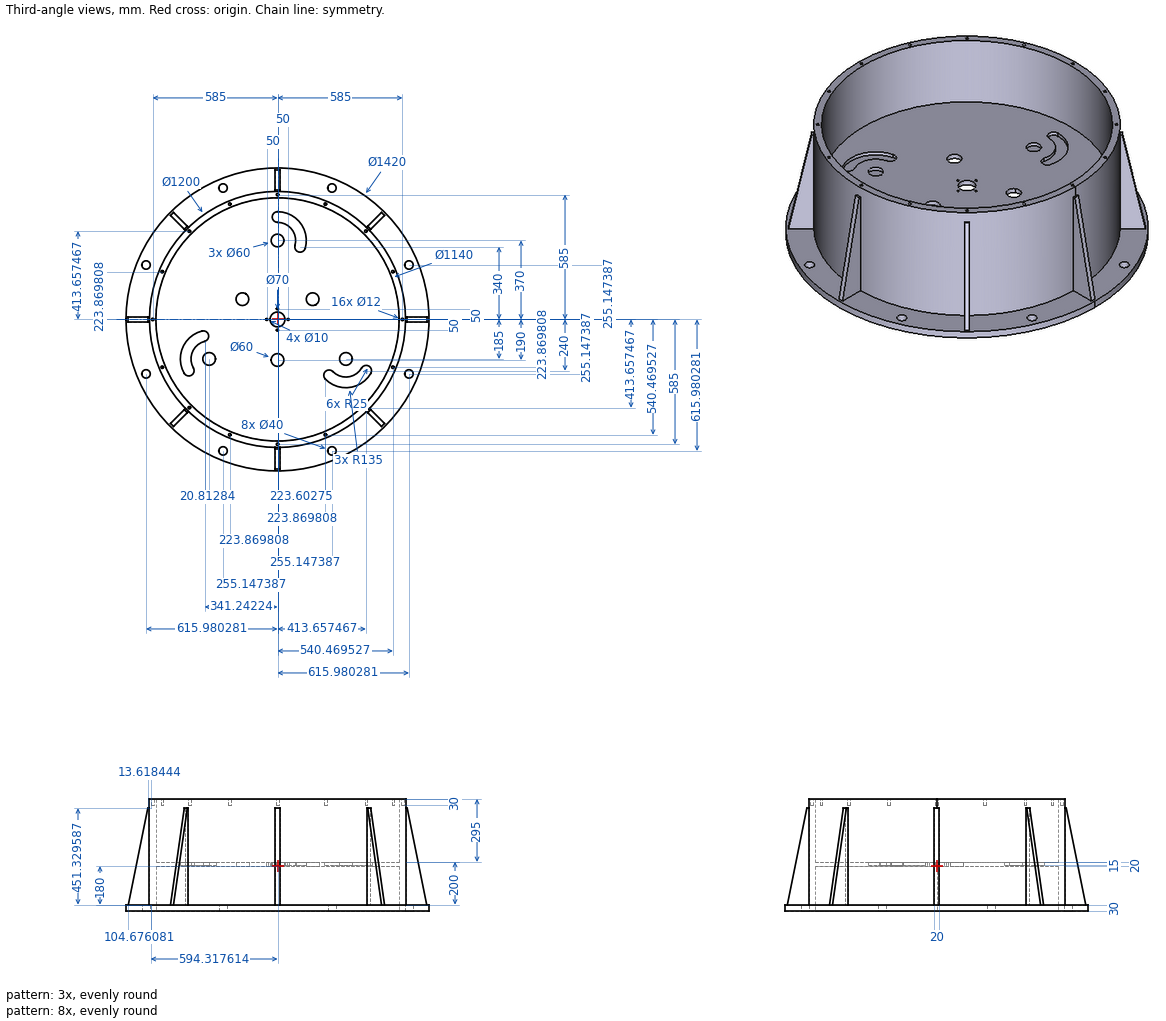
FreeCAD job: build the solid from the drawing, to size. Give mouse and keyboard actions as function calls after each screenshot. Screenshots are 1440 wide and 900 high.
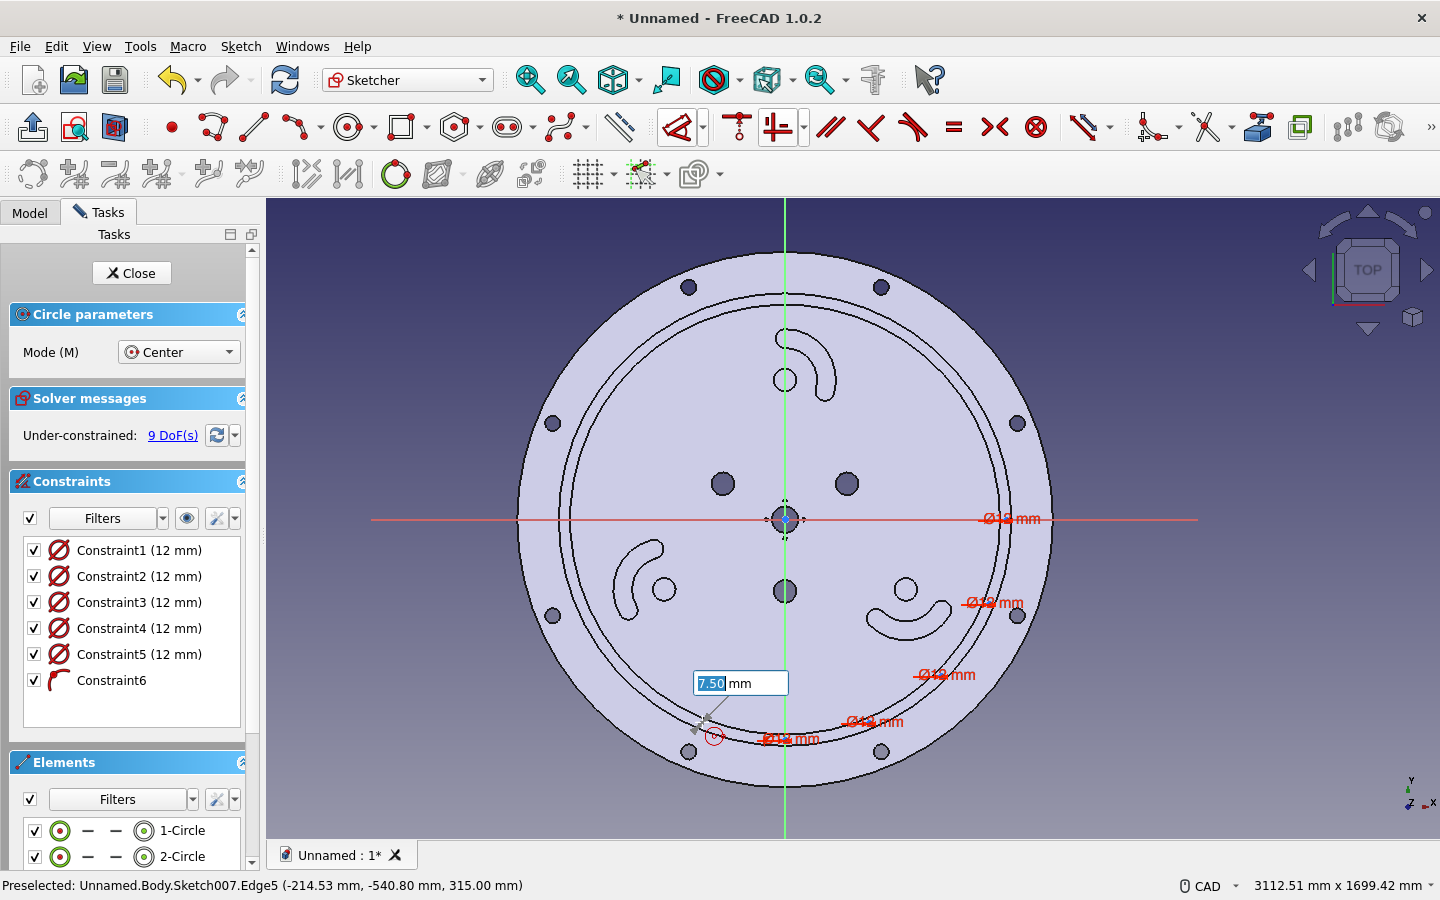
text(12)
key(Return)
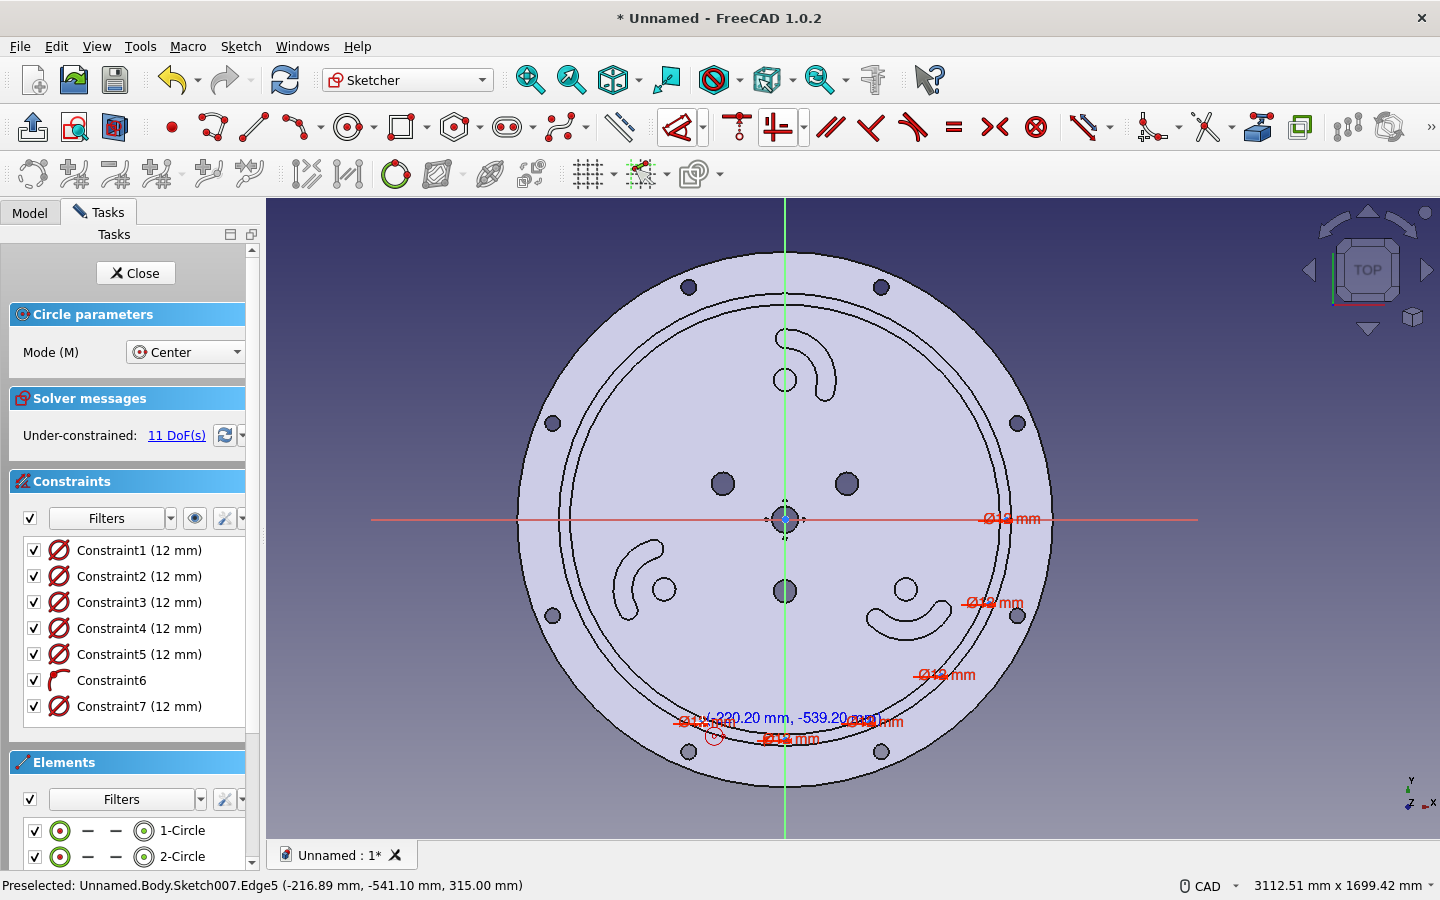
scroll(629, 676, up, 12)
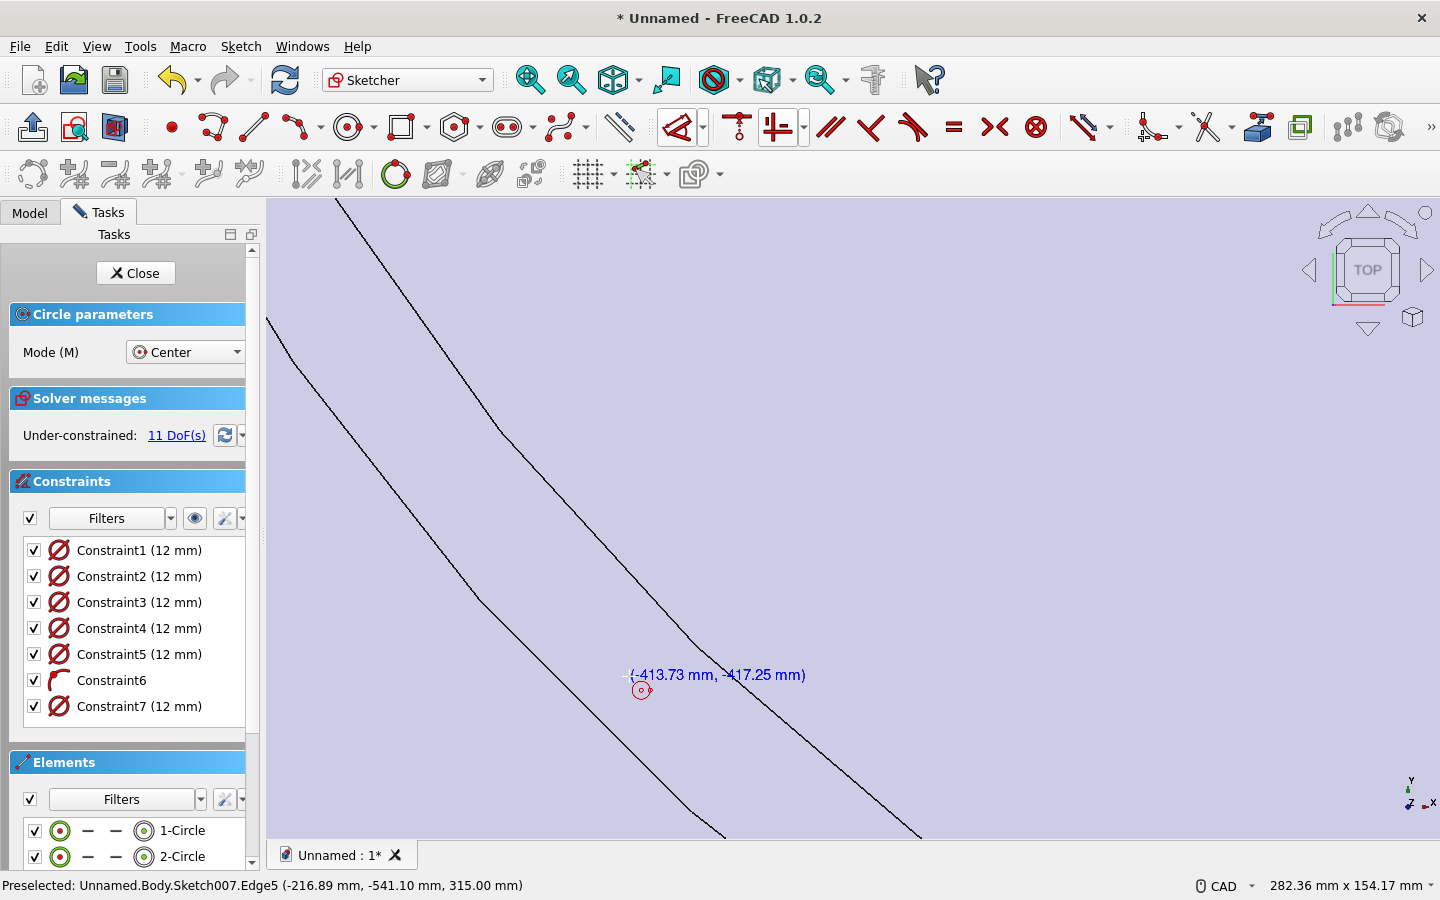
scroll(629, 676, down, 12)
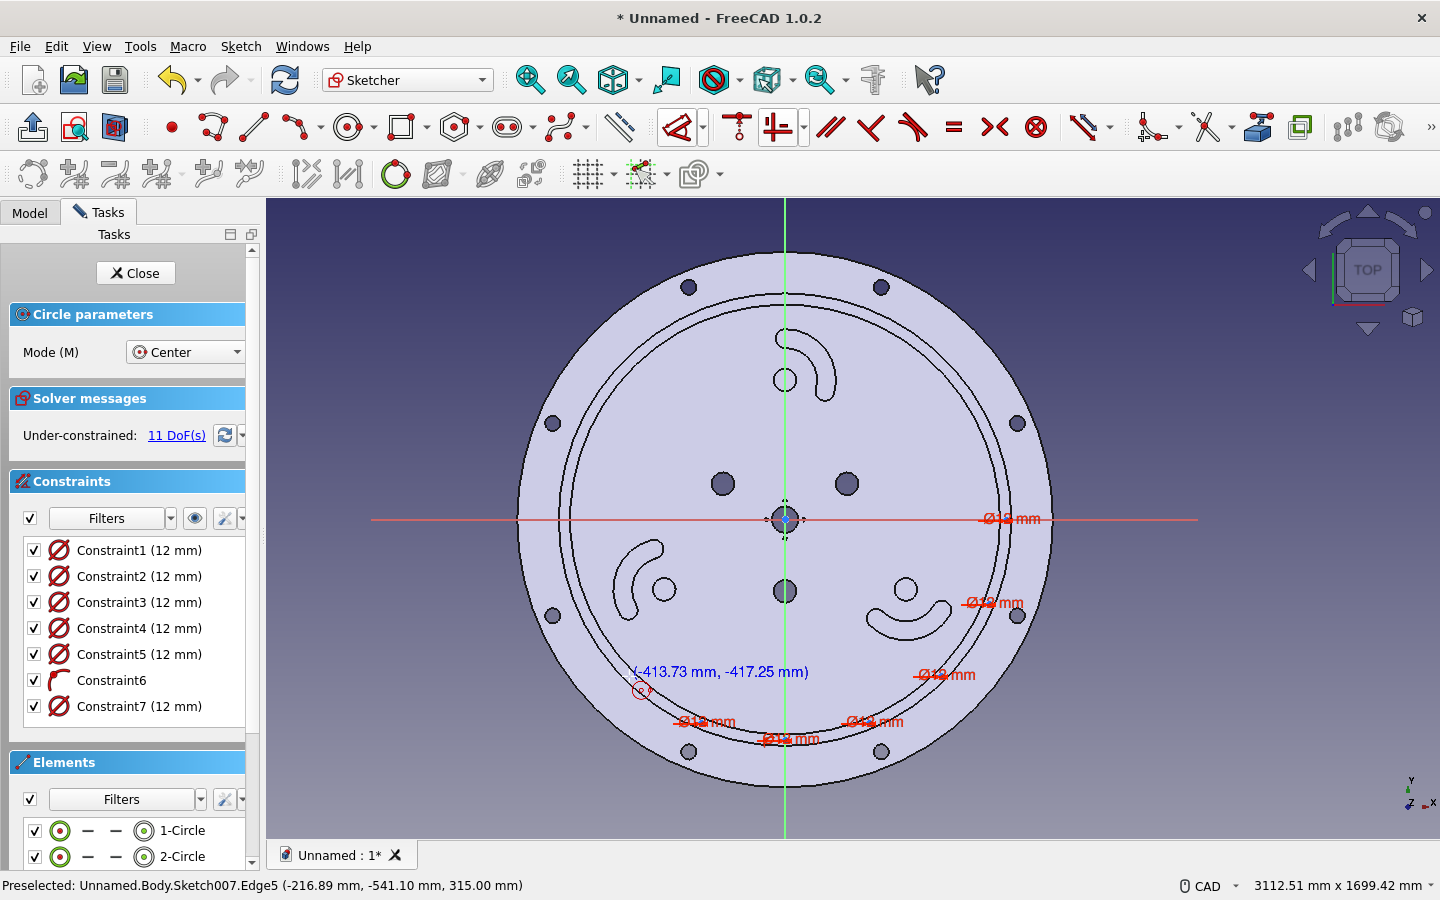
click(629, 676)
move(631, 674)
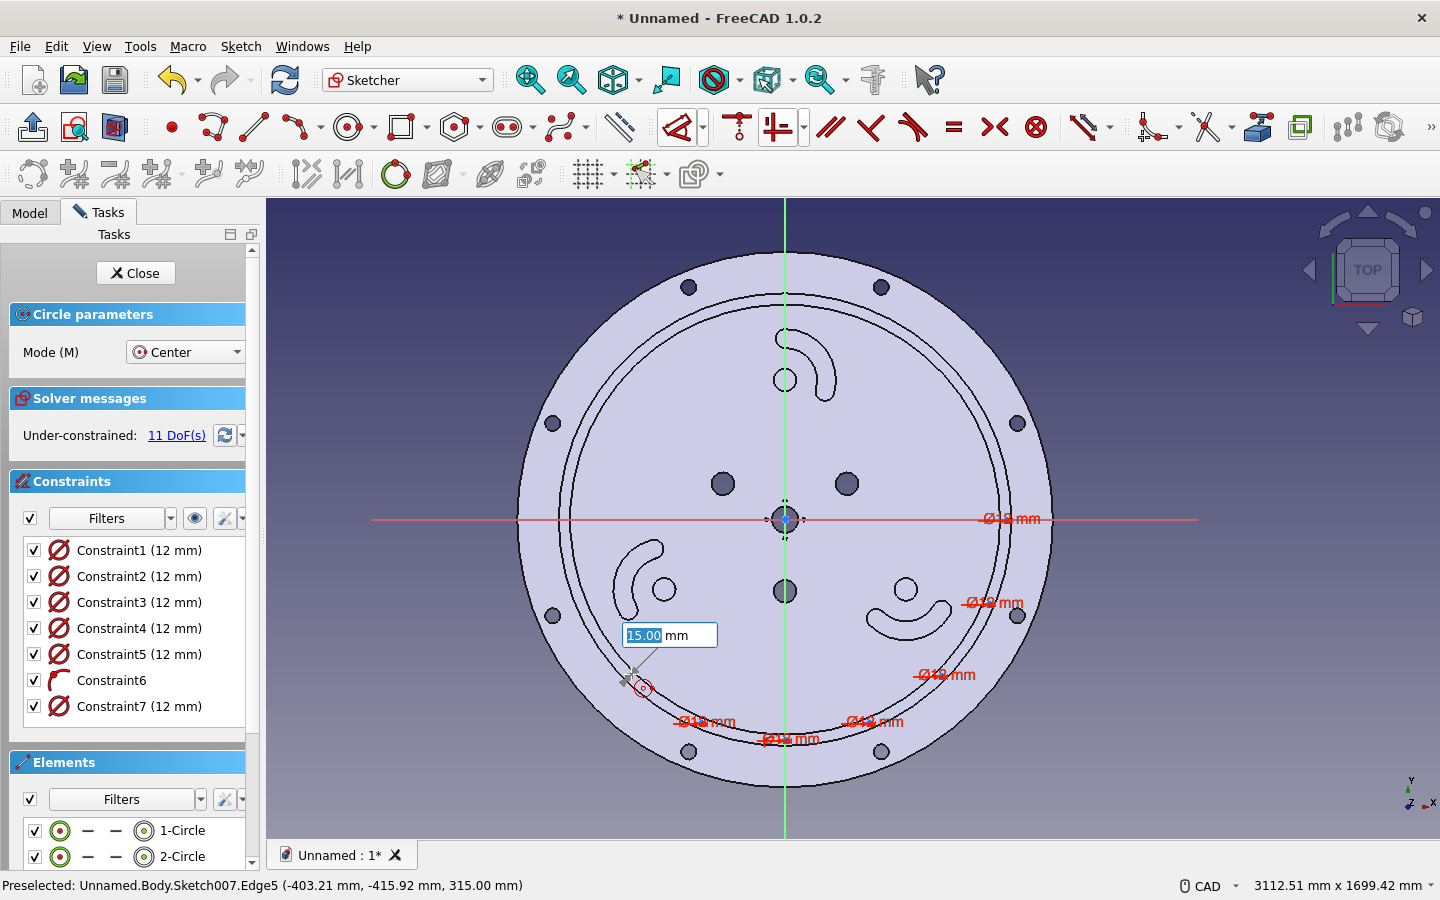
text(12)
key(Return)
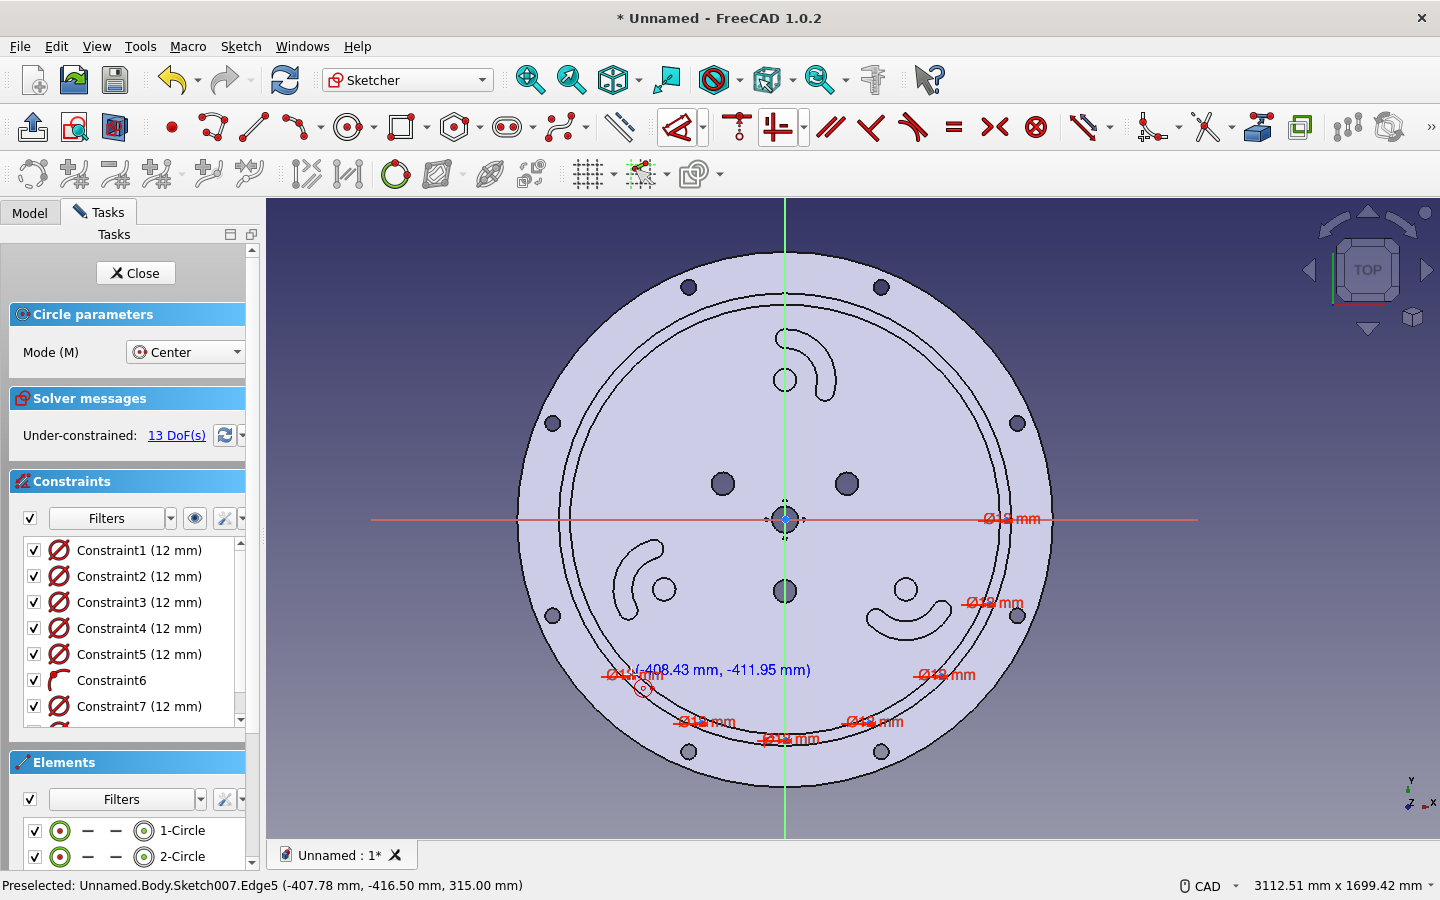
scroll(581, 604, up, 12)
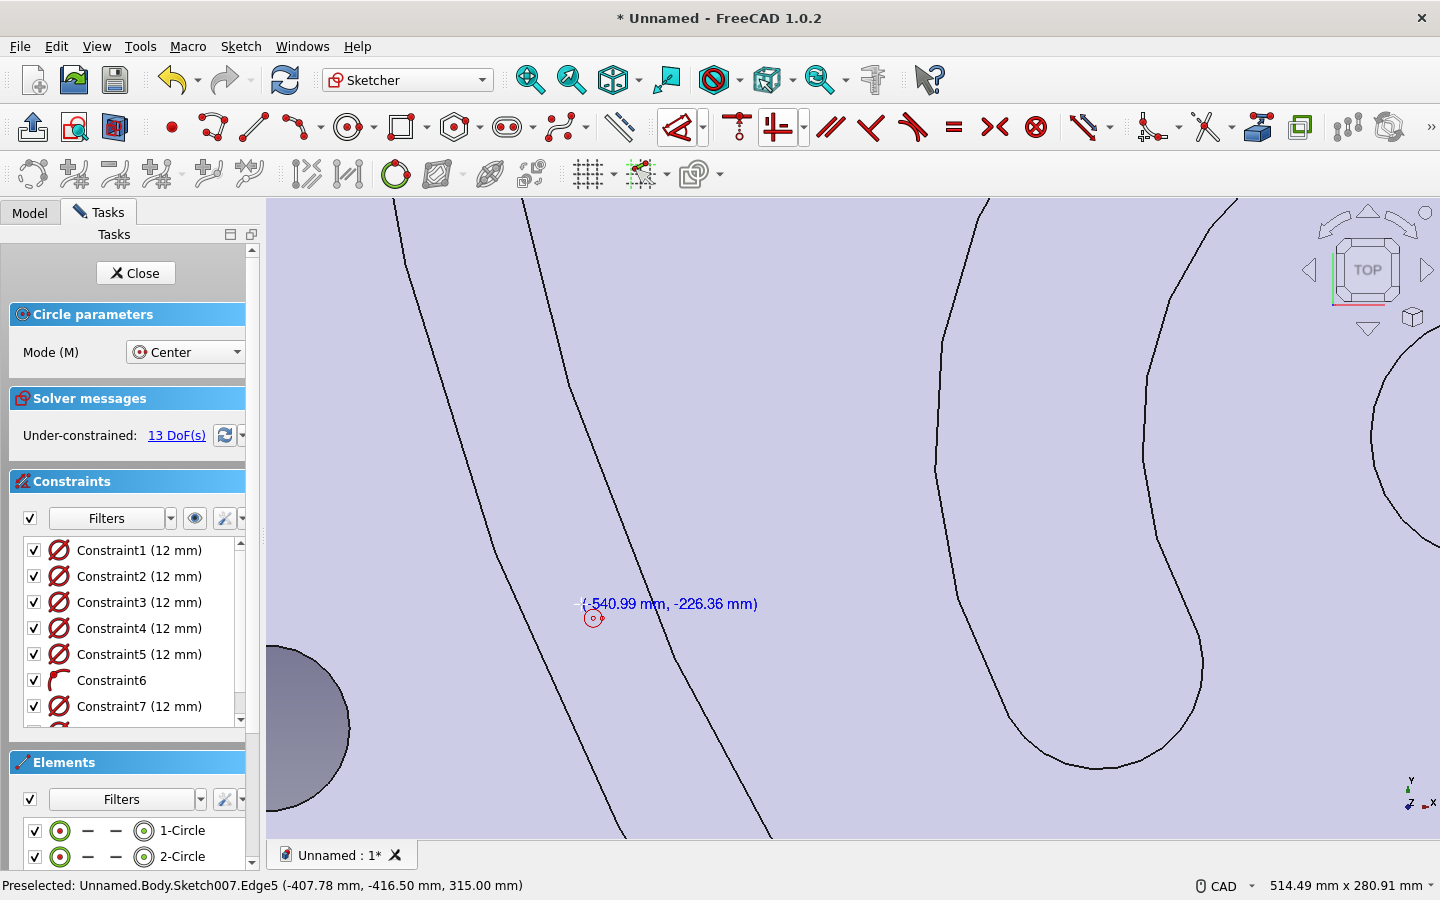
scroll(581, 603, down, 12)